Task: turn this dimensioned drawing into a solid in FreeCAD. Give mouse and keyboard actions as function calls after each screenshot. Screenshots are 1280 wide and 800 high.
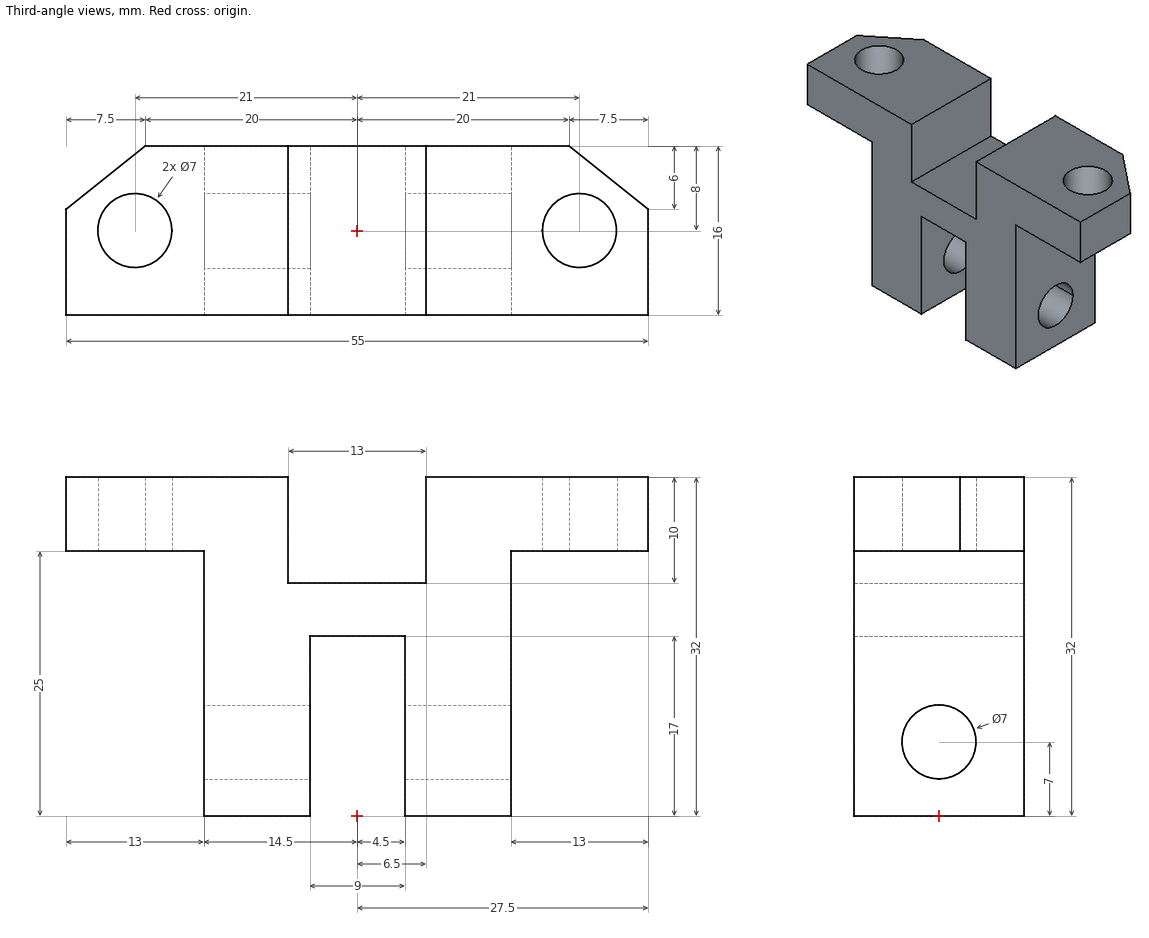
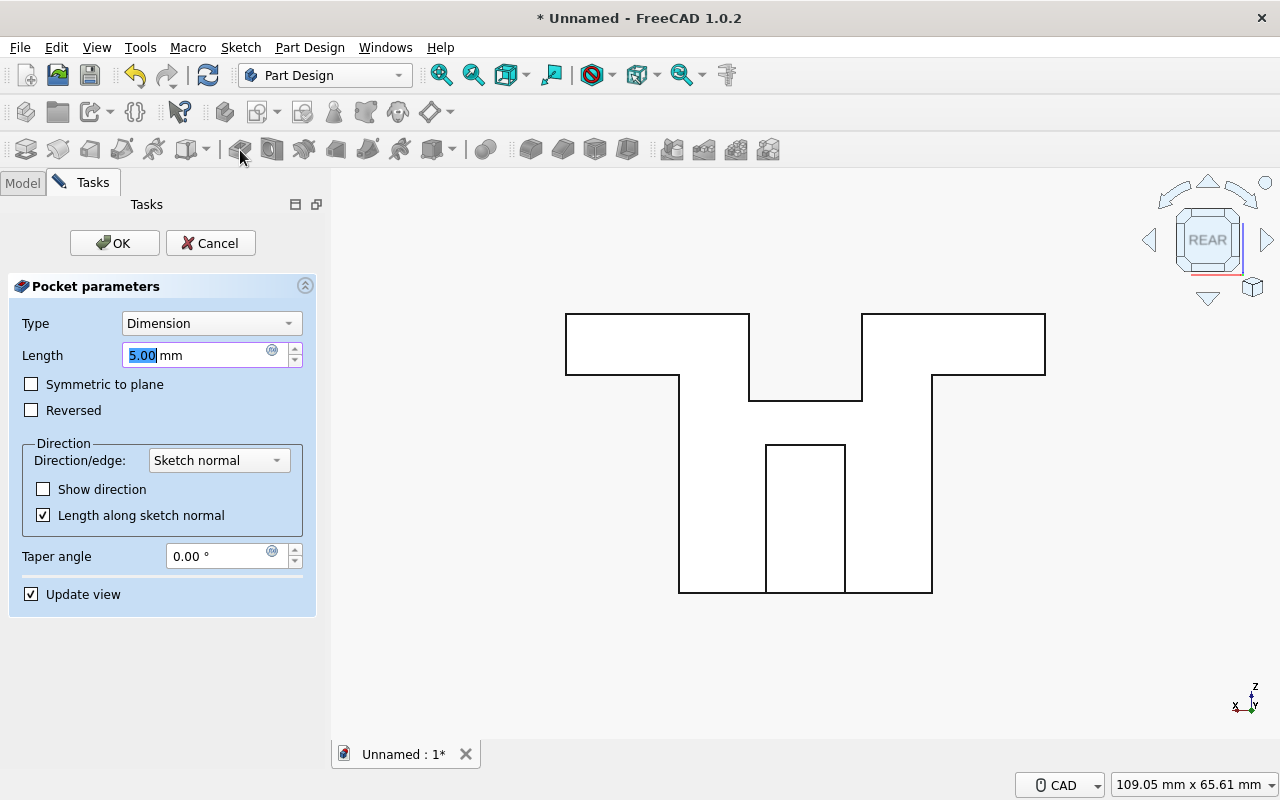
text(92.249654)
key(Tab)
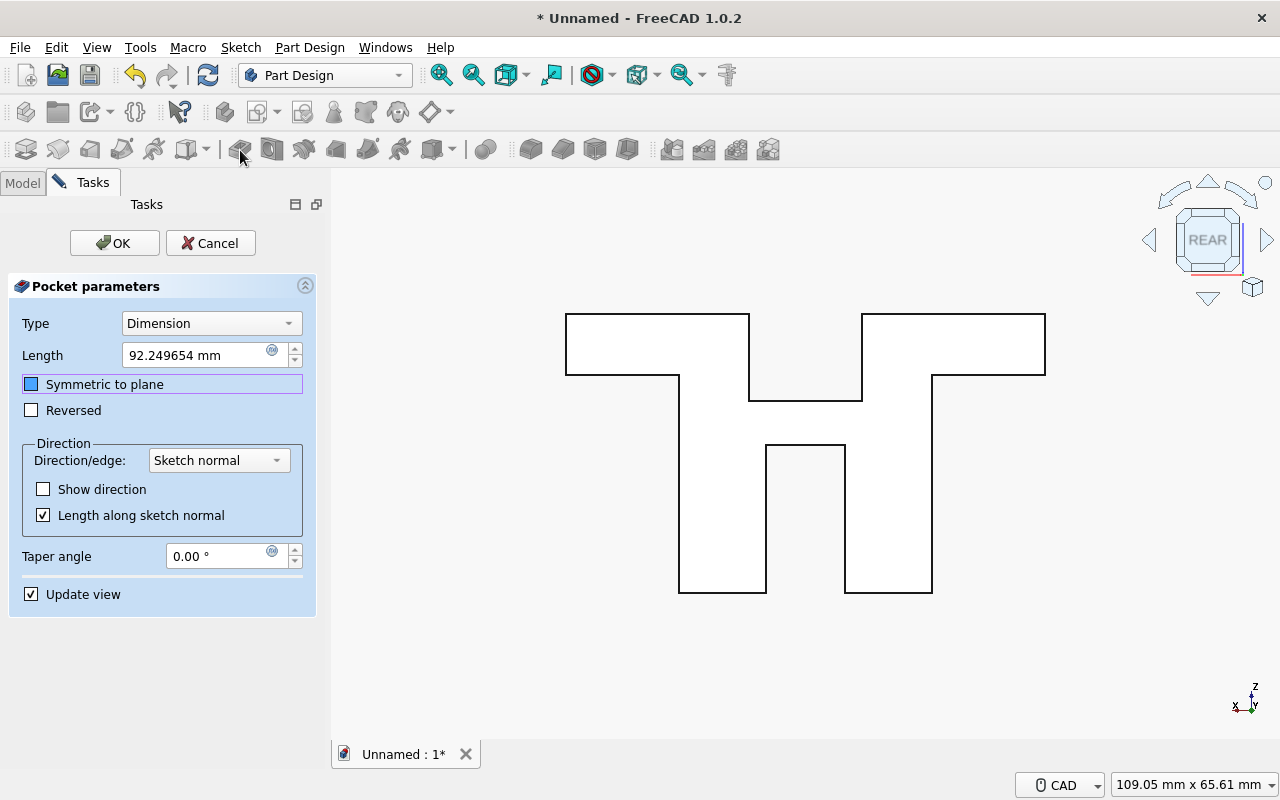
click(30, 384)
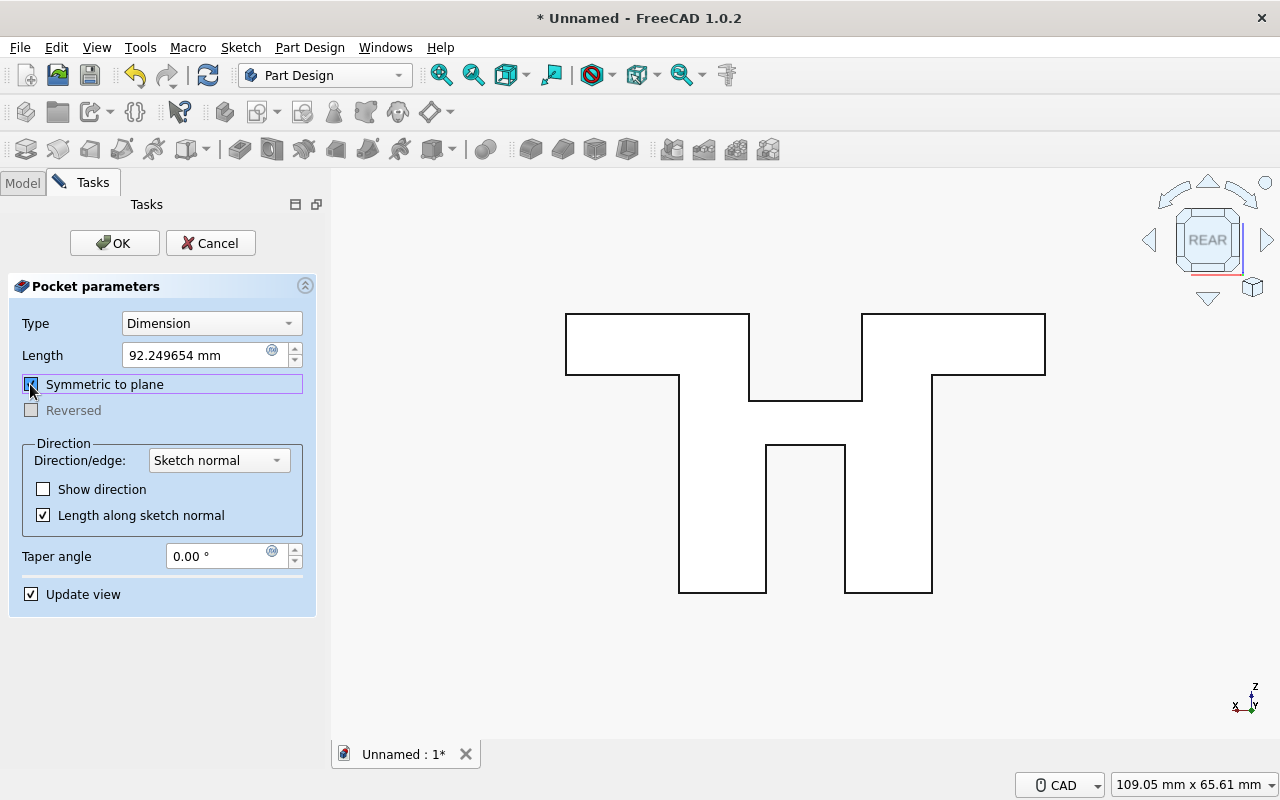
click(115, 243)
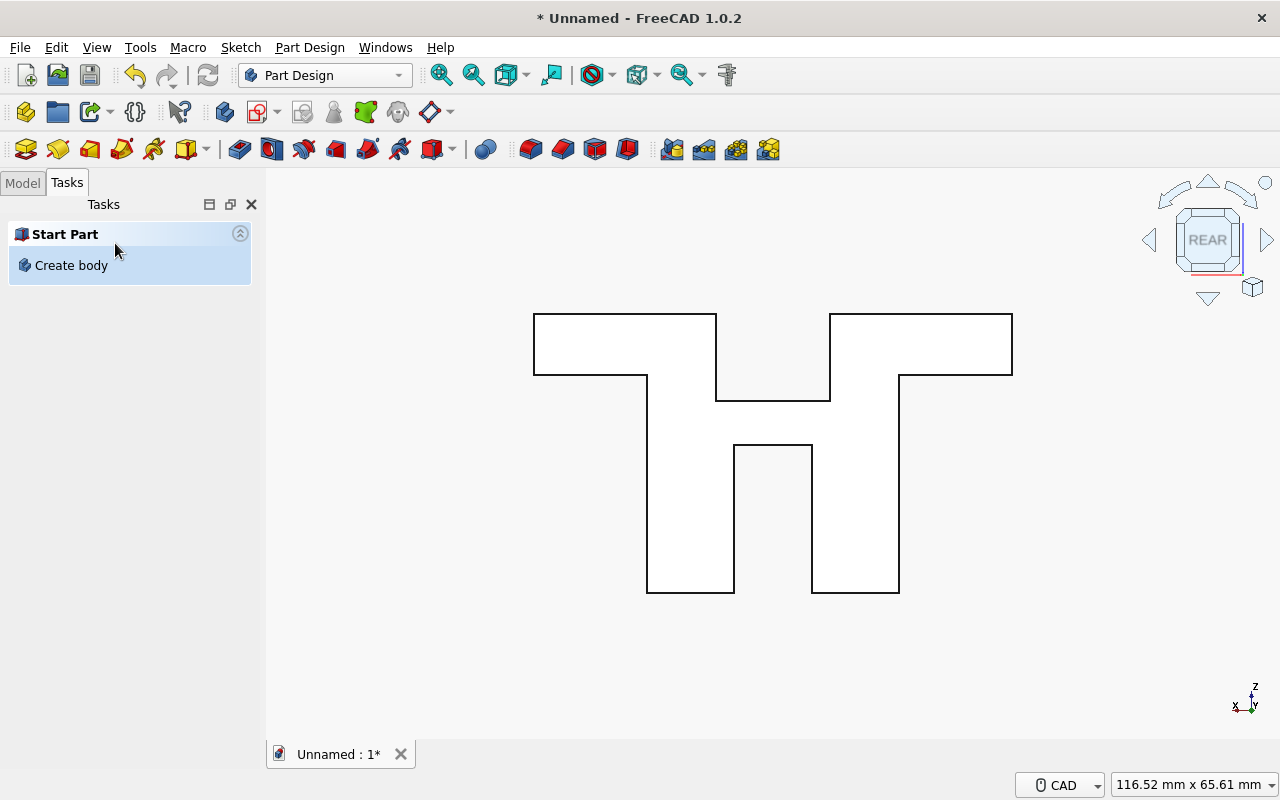
key(5)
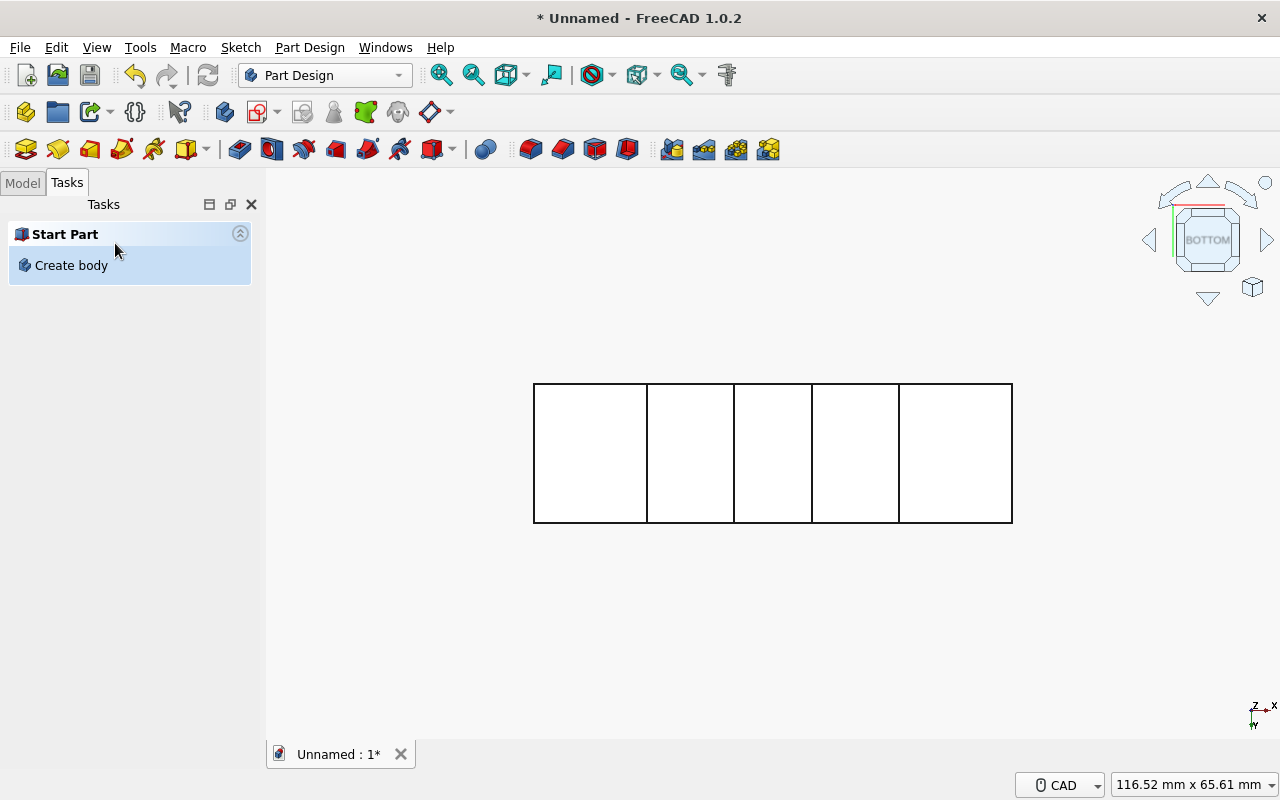
click(590, 453)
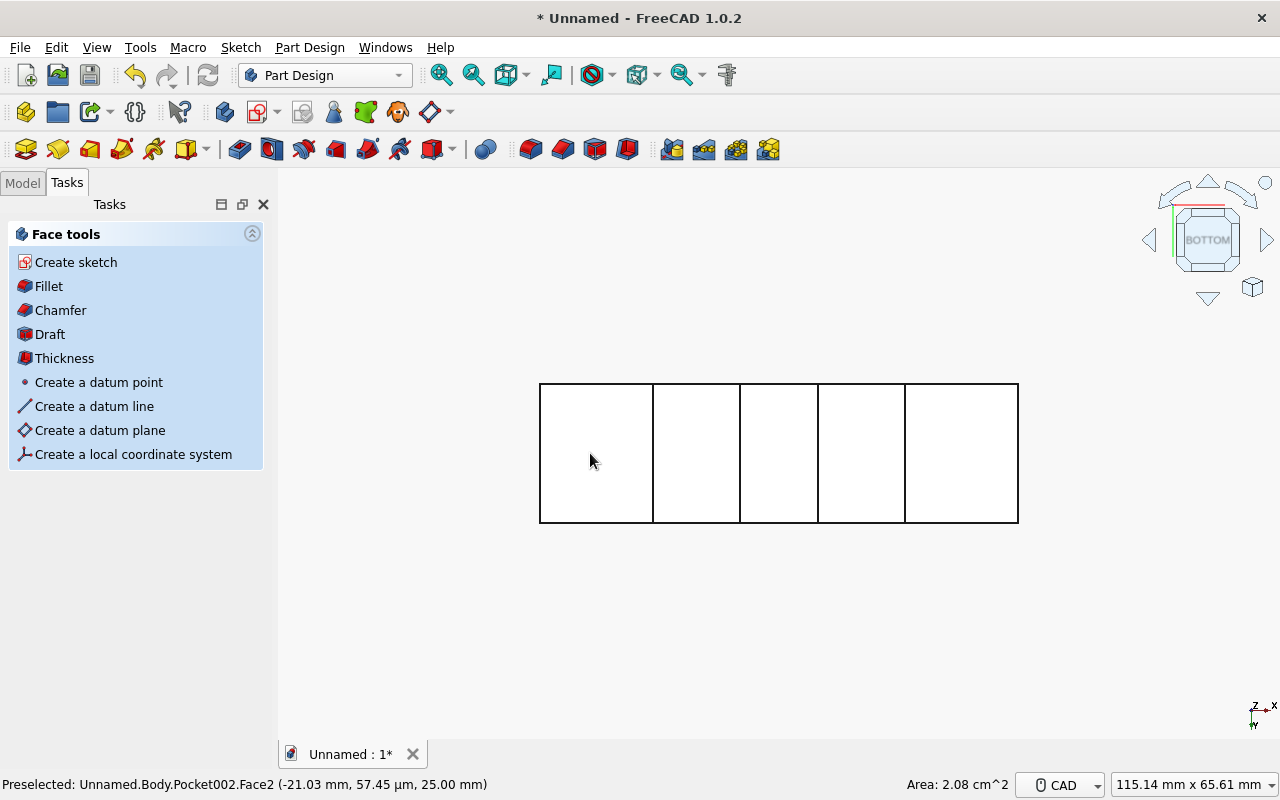
click(258, 112)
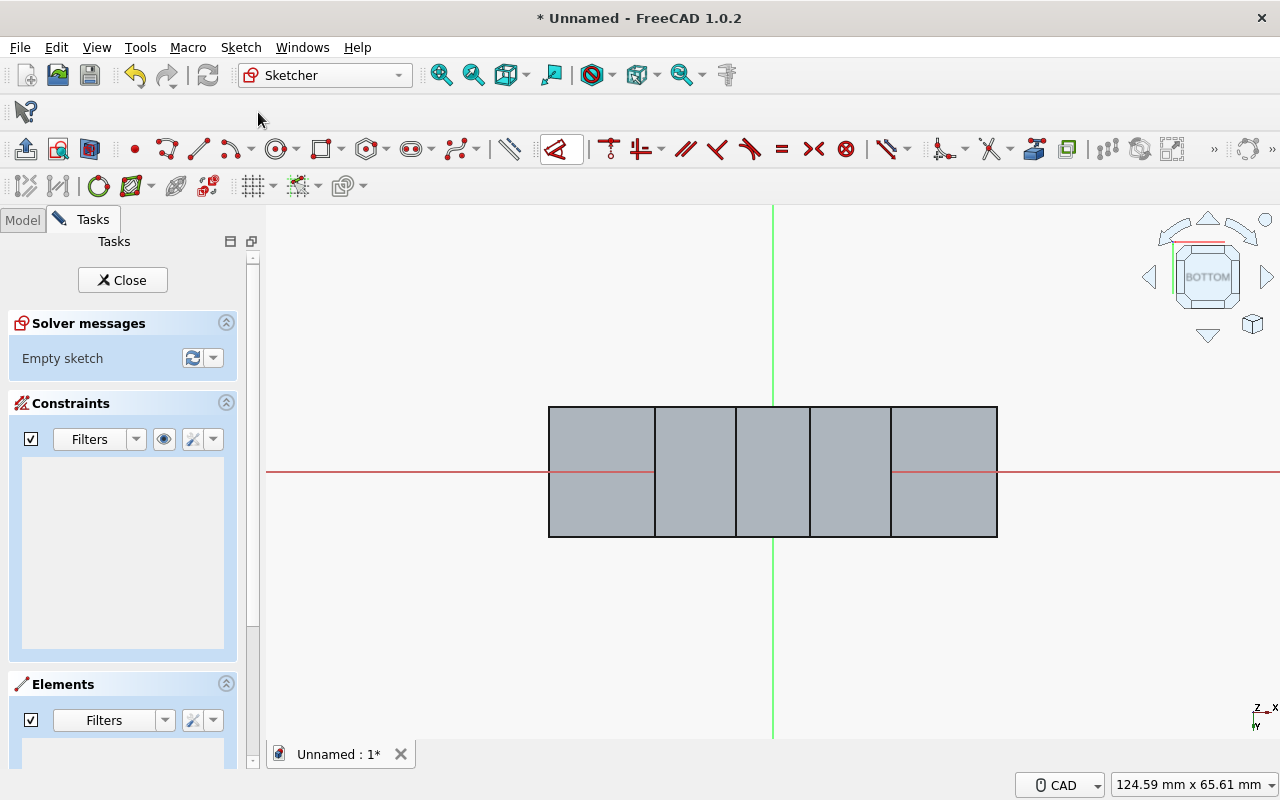
click(168, 150)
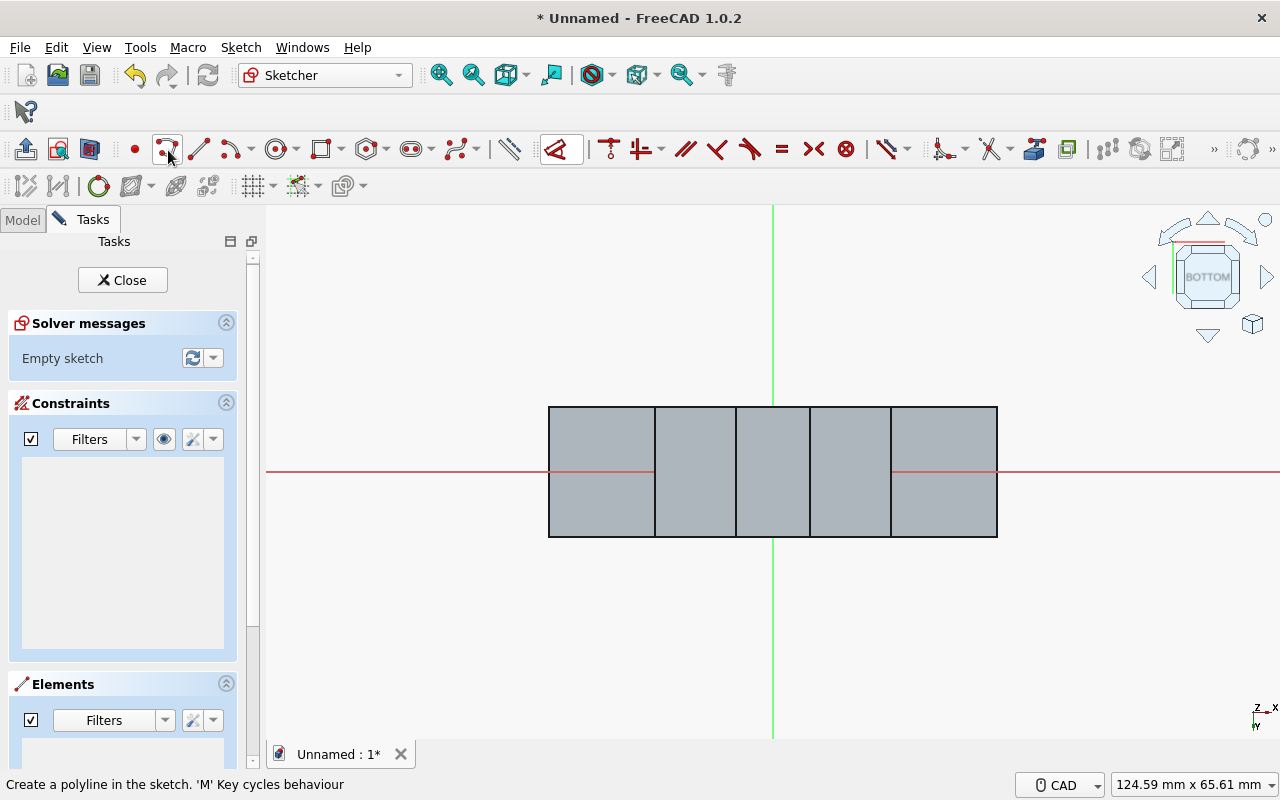
click(936, 537)
click(997, 537)
click(997, 488)
click(936, 538)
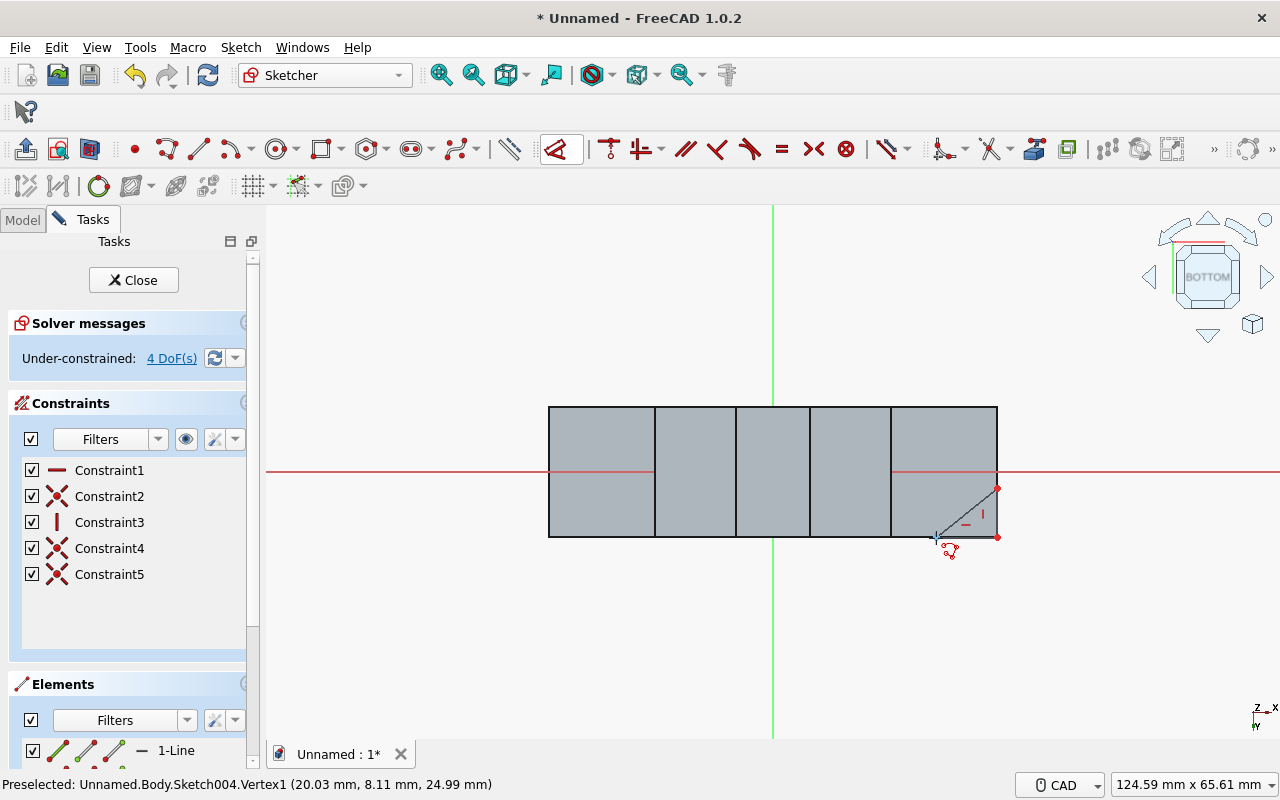
click(610, 537)
click(549, 488)
click(549, 537)
click(610, 538)
key(Escape)
key(Escape)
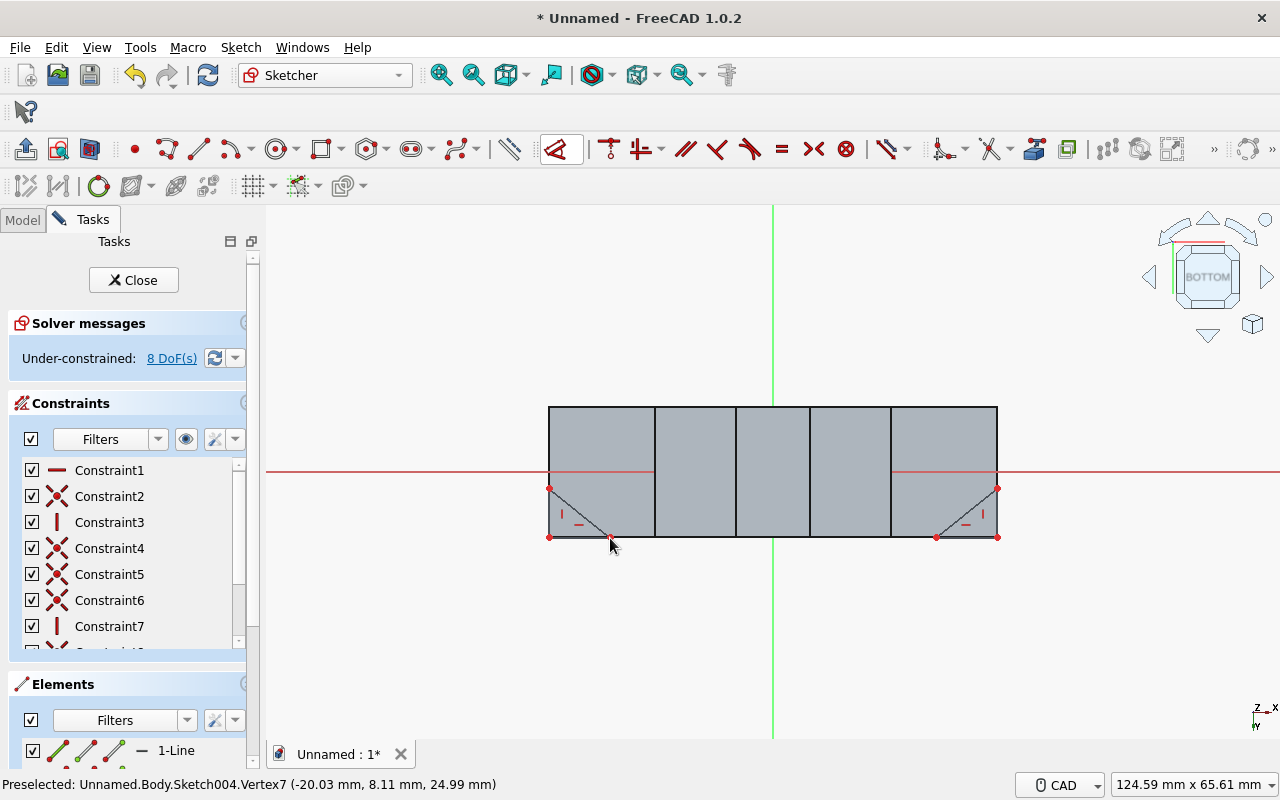
click(997, 523)